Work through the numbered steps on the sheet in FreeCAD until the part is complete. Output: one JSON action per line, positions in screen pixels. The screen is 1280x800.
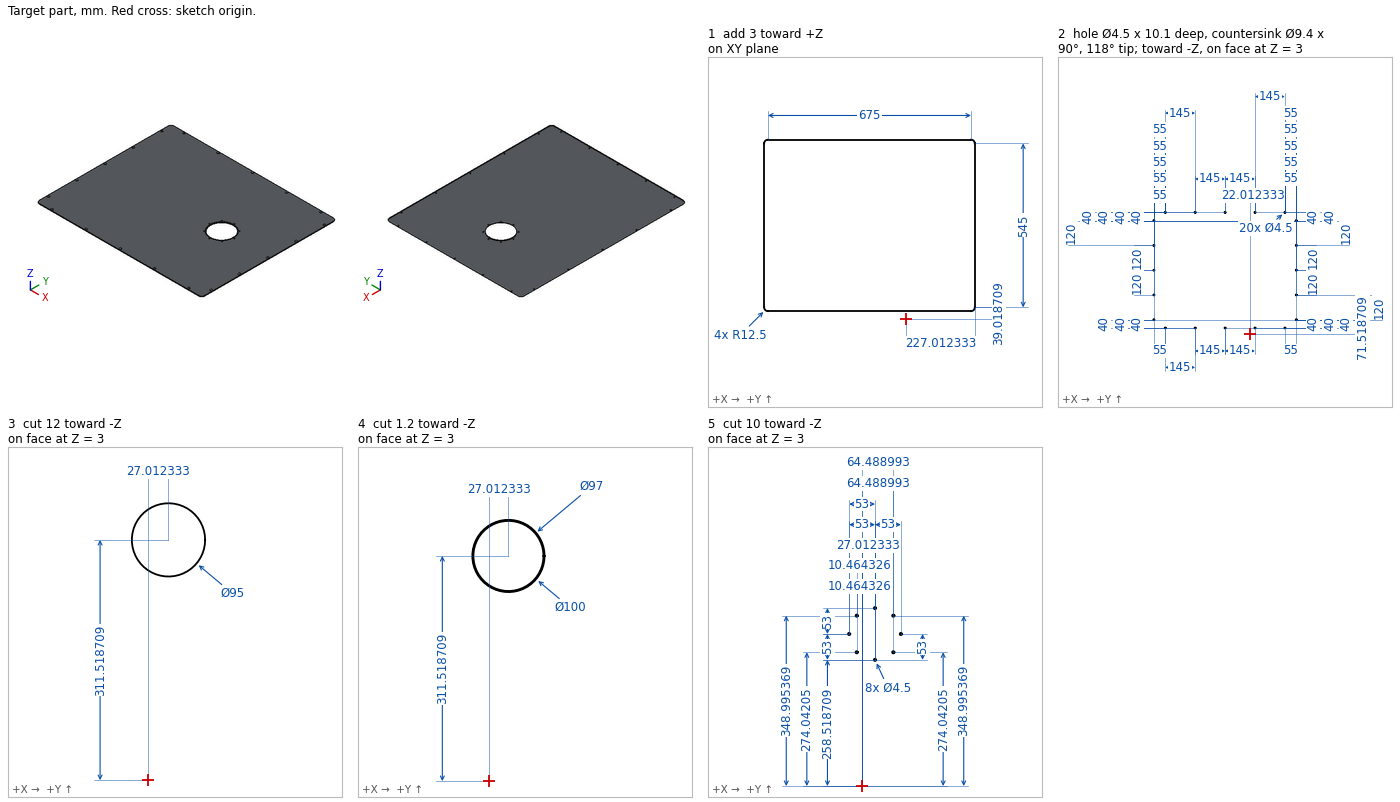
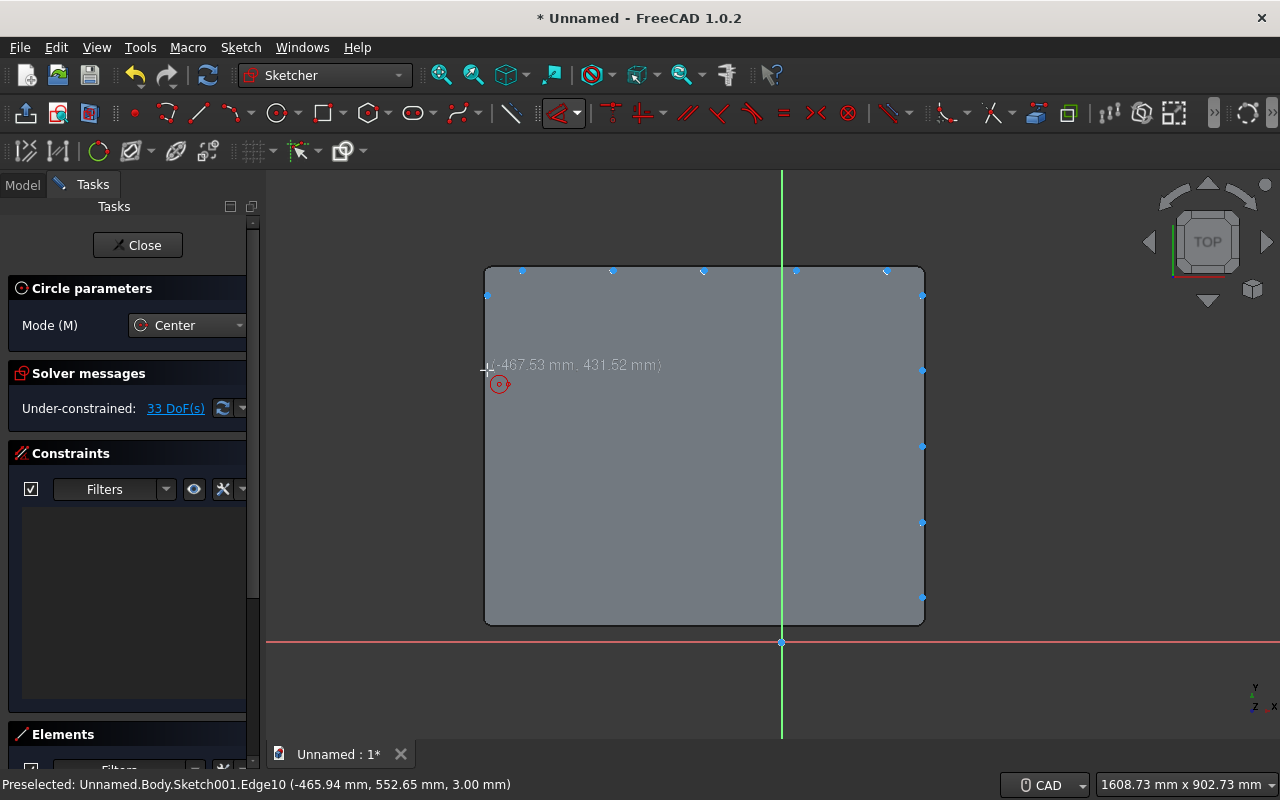
{"action": "left_click", "coordinate": [487, 370]}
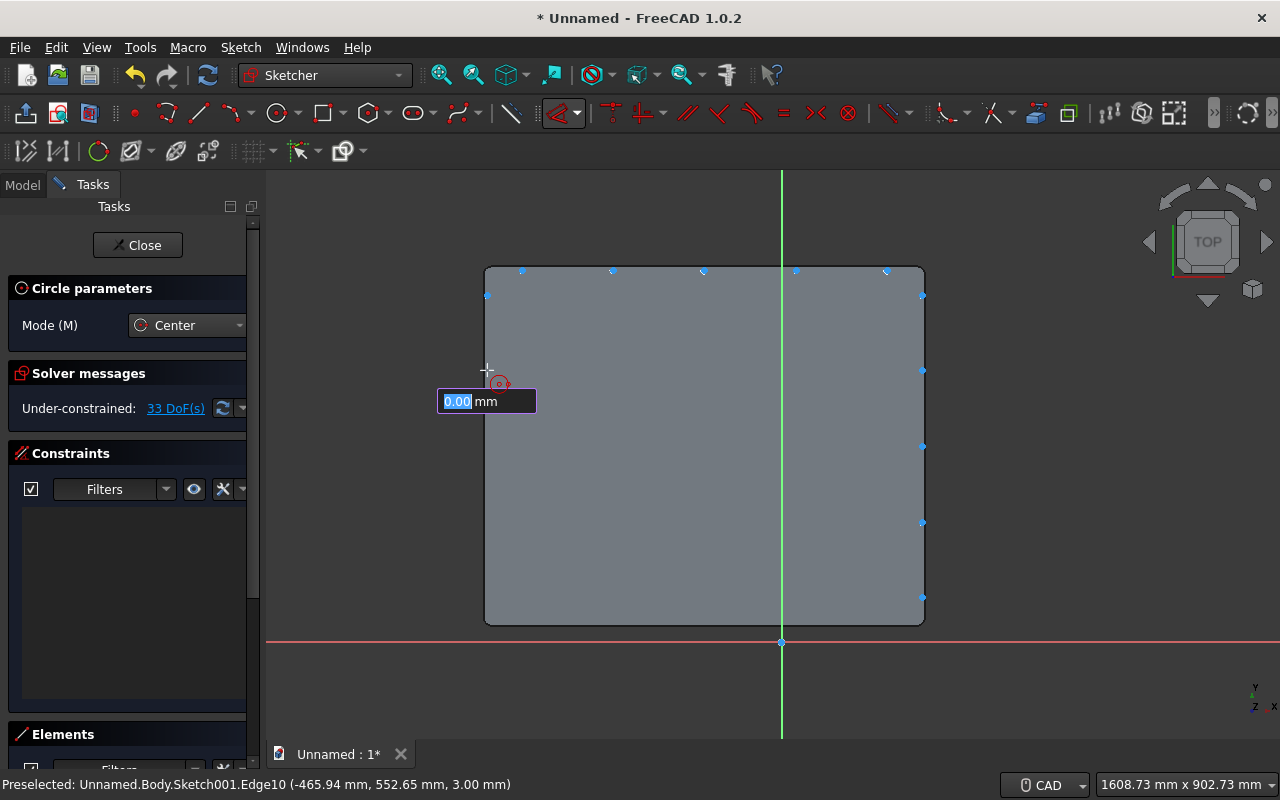
{"action": "scroll", "coordinate": [488, 369], "scroll_direction": "up", "scroll_amount": 13}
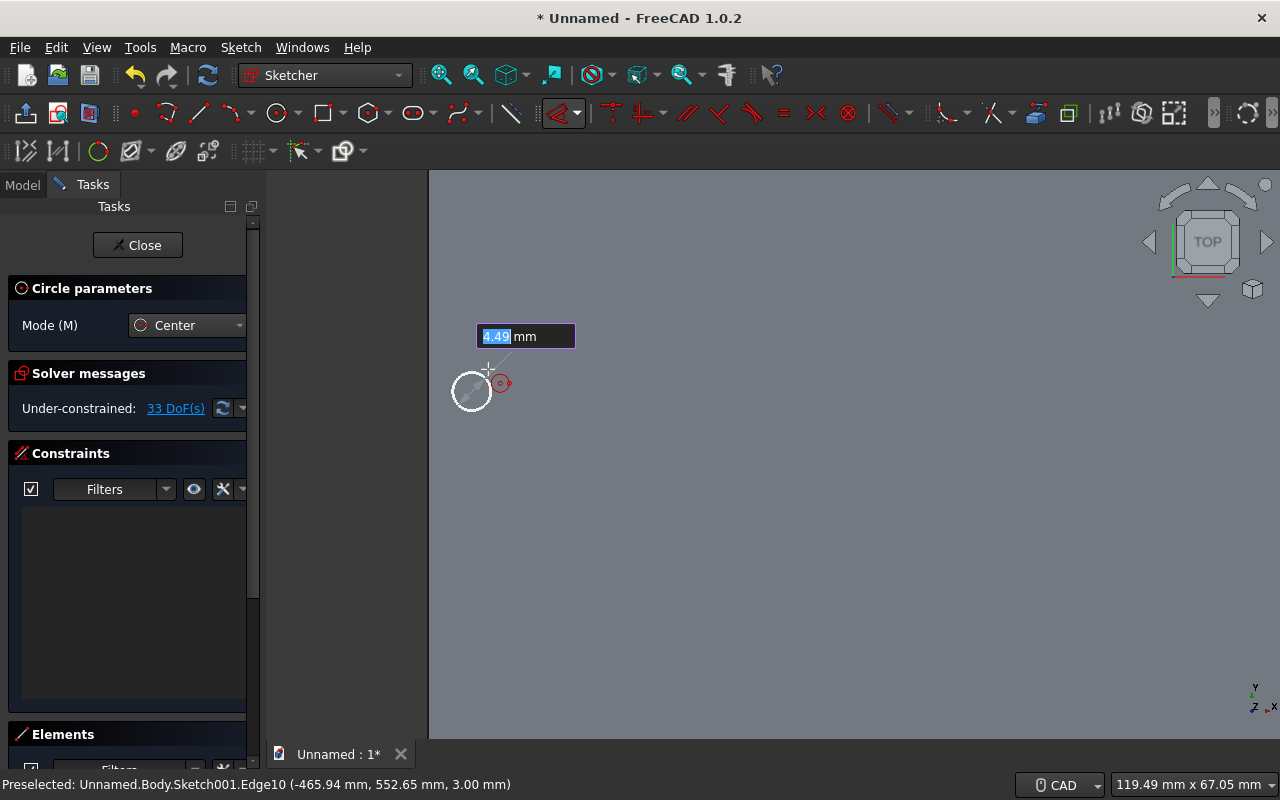
{"action": "left_click", "coordinate": [484, 370]}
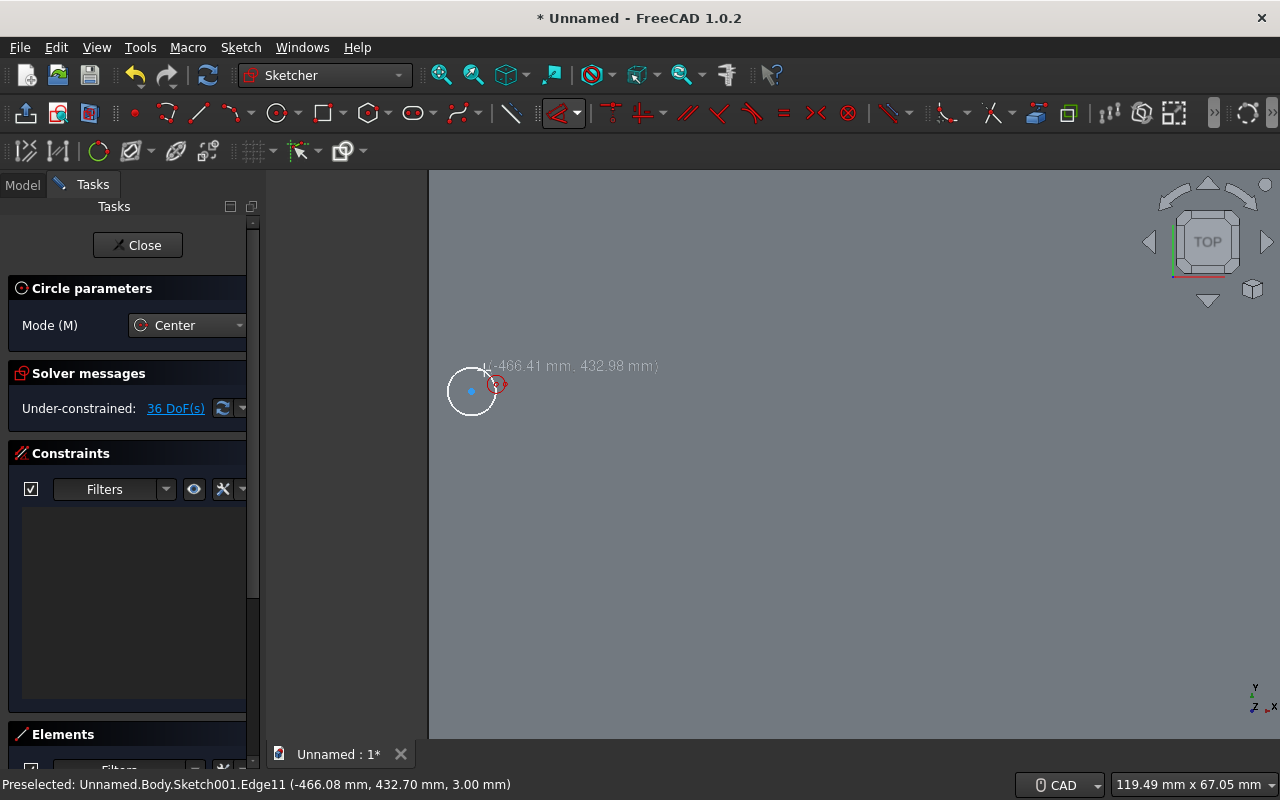
{"action": "scroll", "coordinate": [488, 369], "scroll_direction": "down", "scroll_amount": 13}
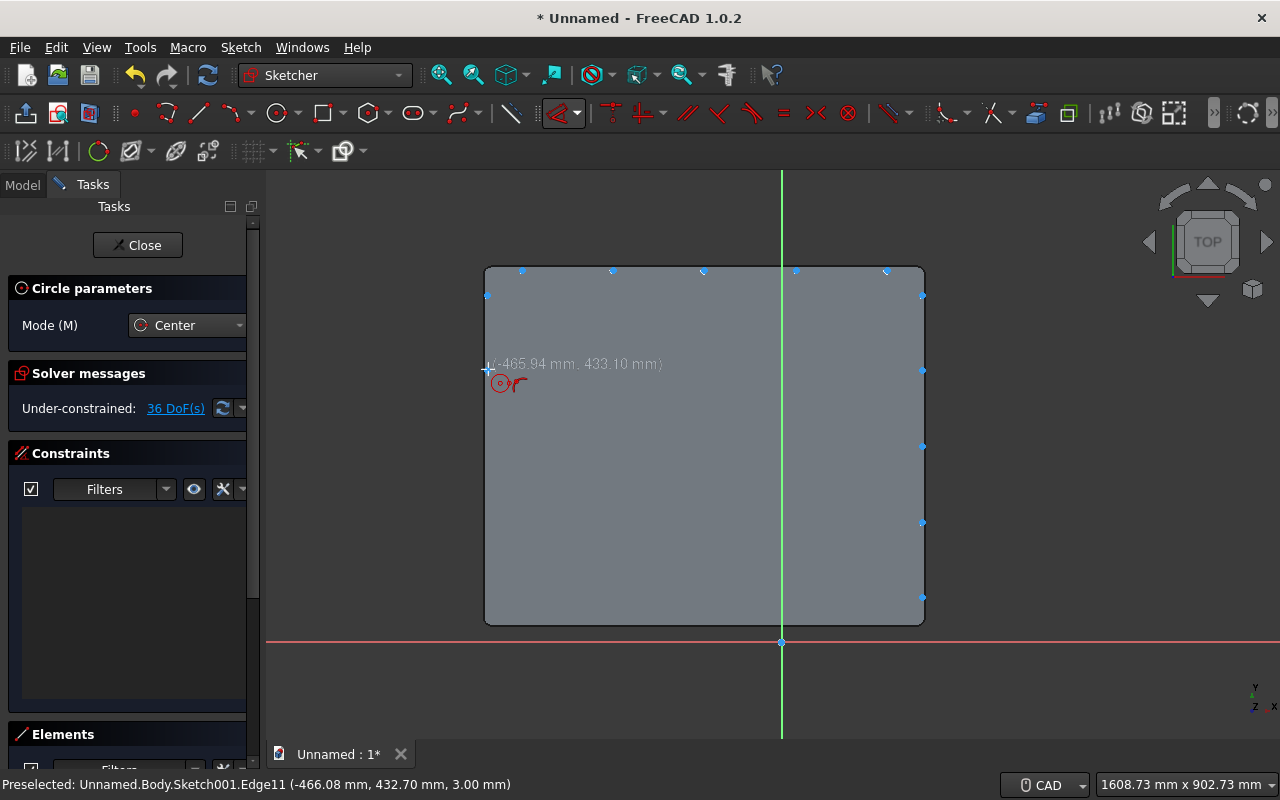
{"action": "scroll", "coordinate": [487, 446], "scroll_direction": "up", "scroll_amount": 14}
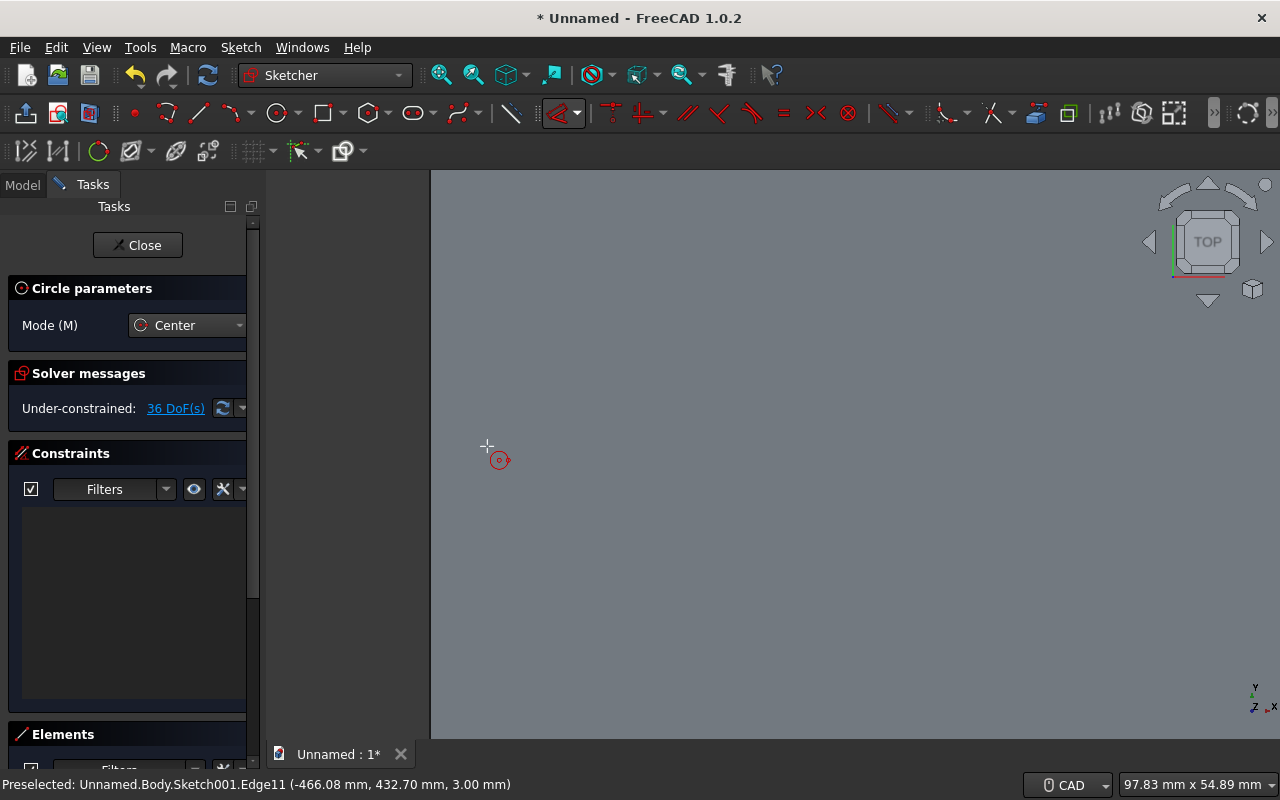
{"action": "scroll", "coordinate": [487, 446], "scroll_direction": "down", "scroll_amount": 14}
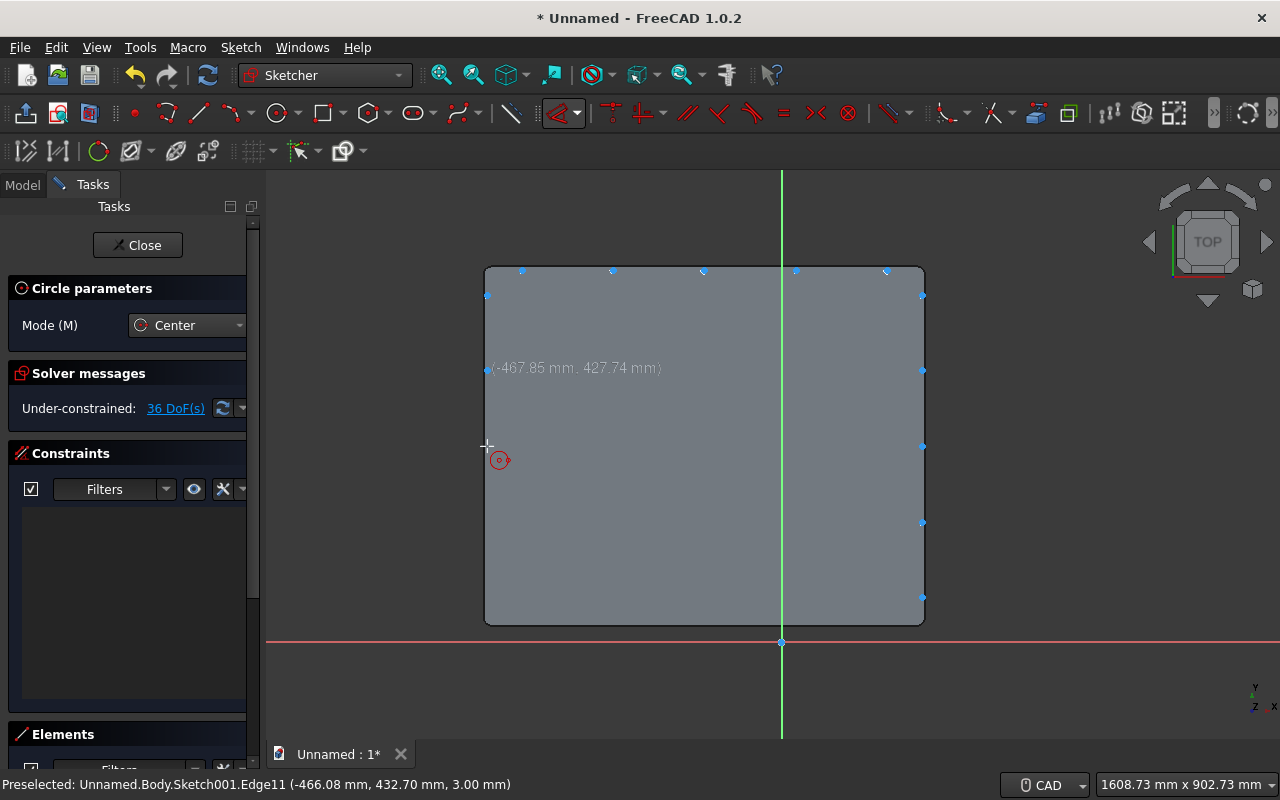
{"action": "left_click", "coordinate": [487, 446]}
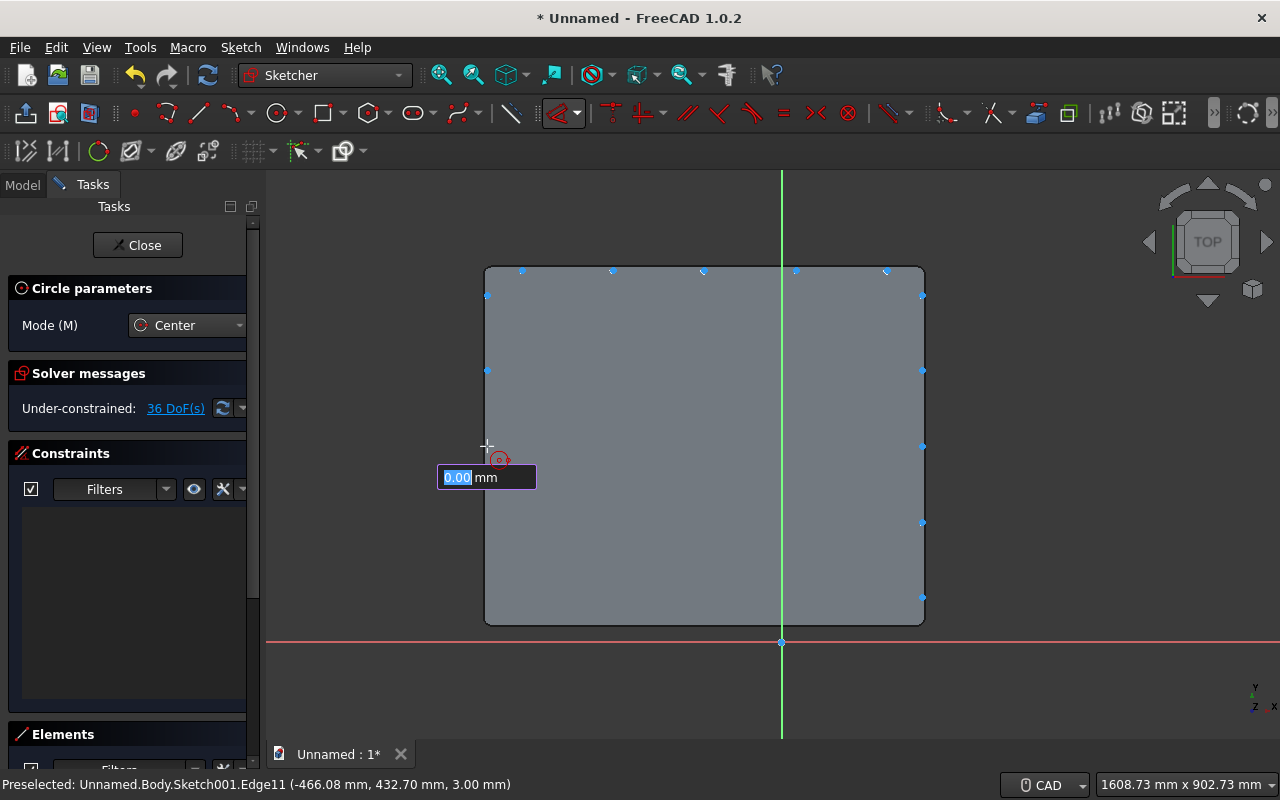
{"action": "scroll", "coordinate": [488, 445], "scroll_direction": "up", "scroll_amount": 13}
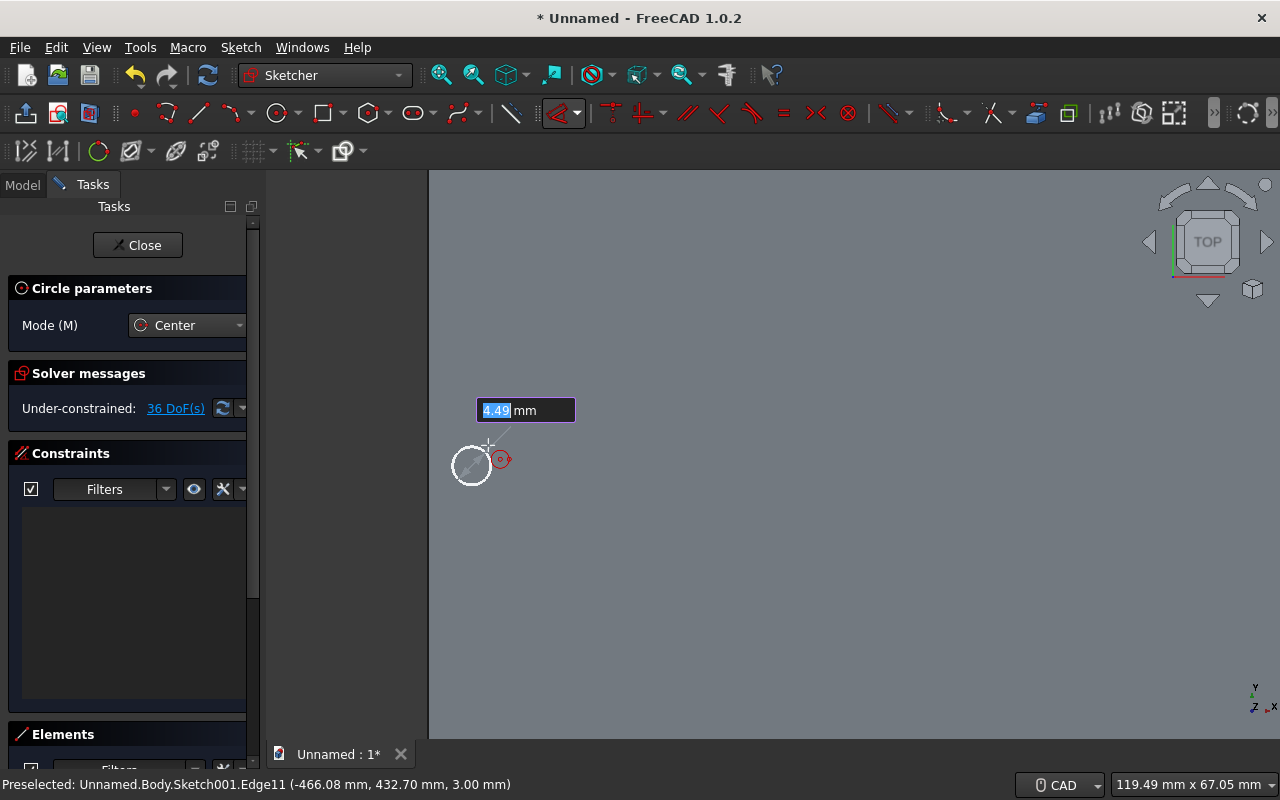
{"action": "left_click", "coordinate": [484, 439]}